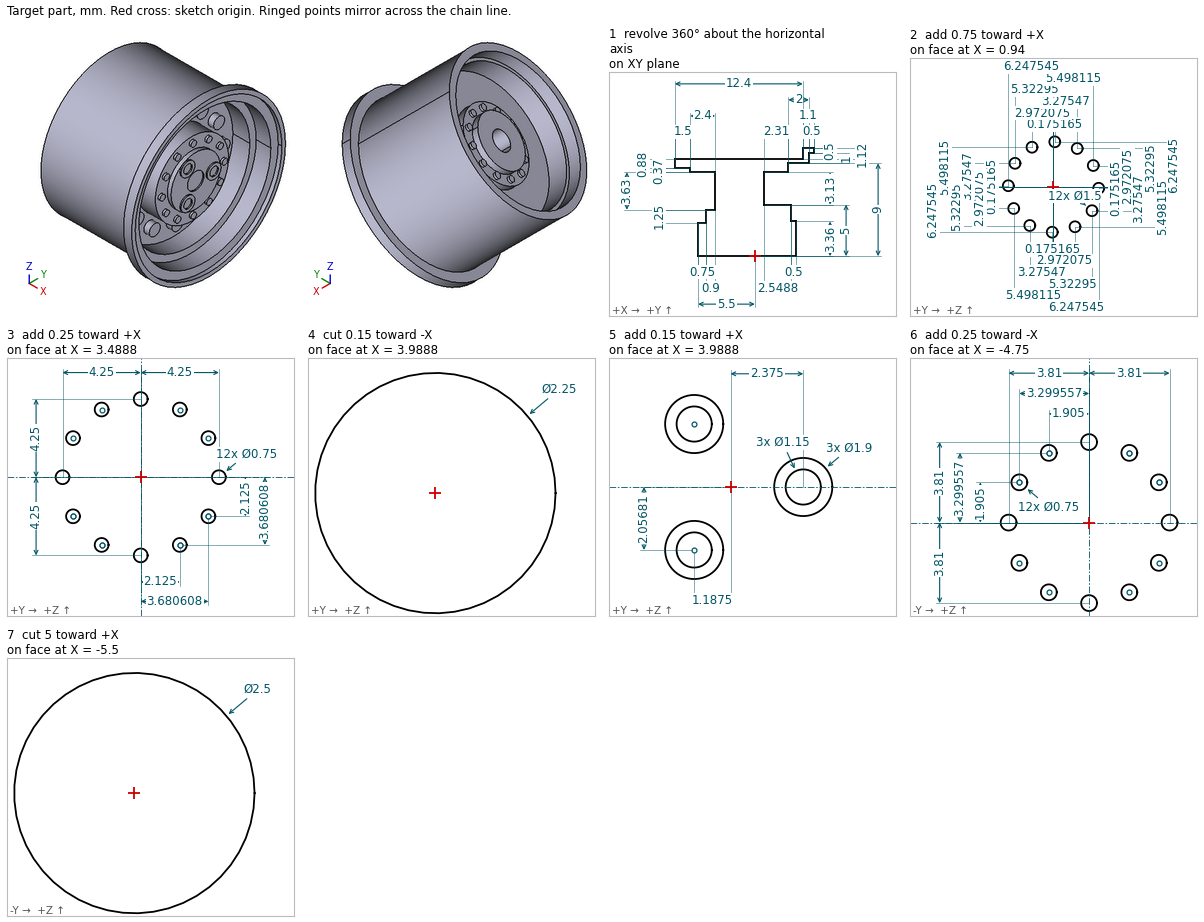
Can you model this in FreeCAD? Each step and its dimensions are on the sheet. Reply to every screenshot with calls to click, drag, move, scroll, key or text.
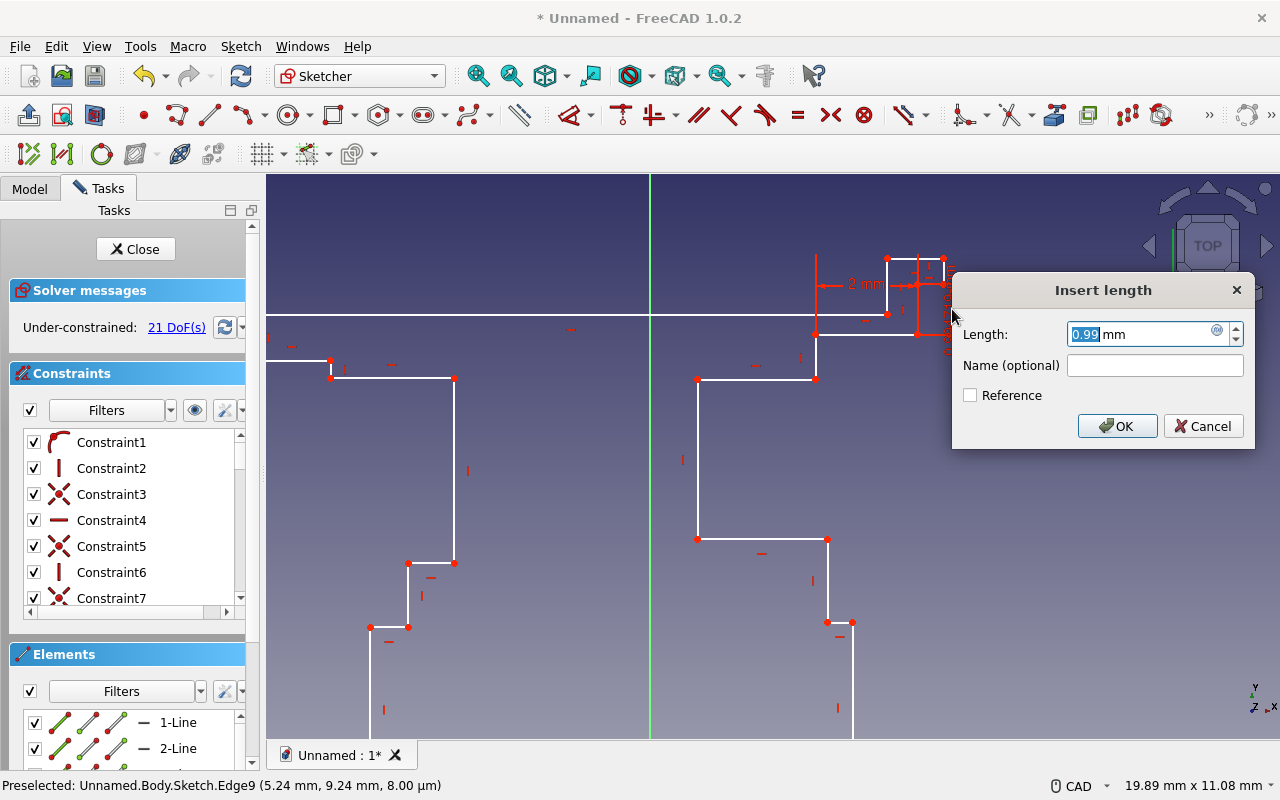
text(1)
key(Return)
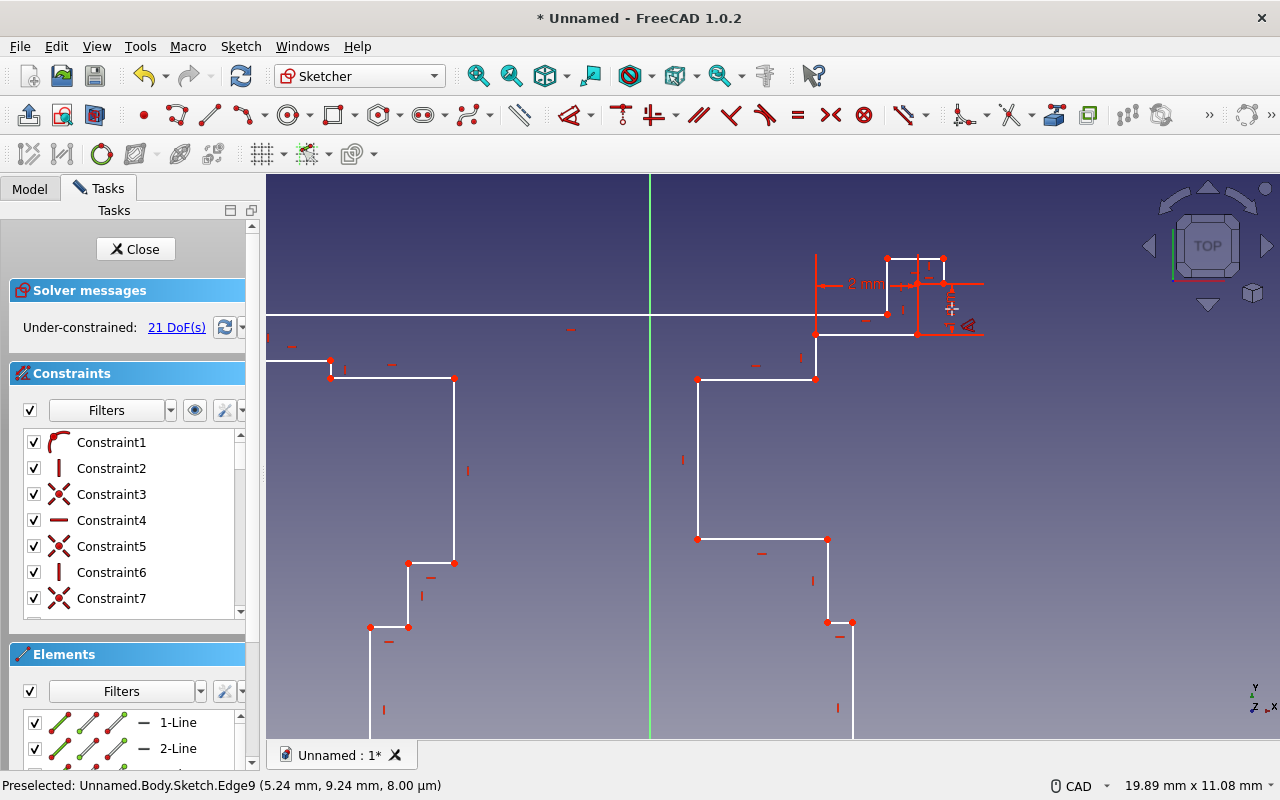
click(828, 539)
click(862, 586)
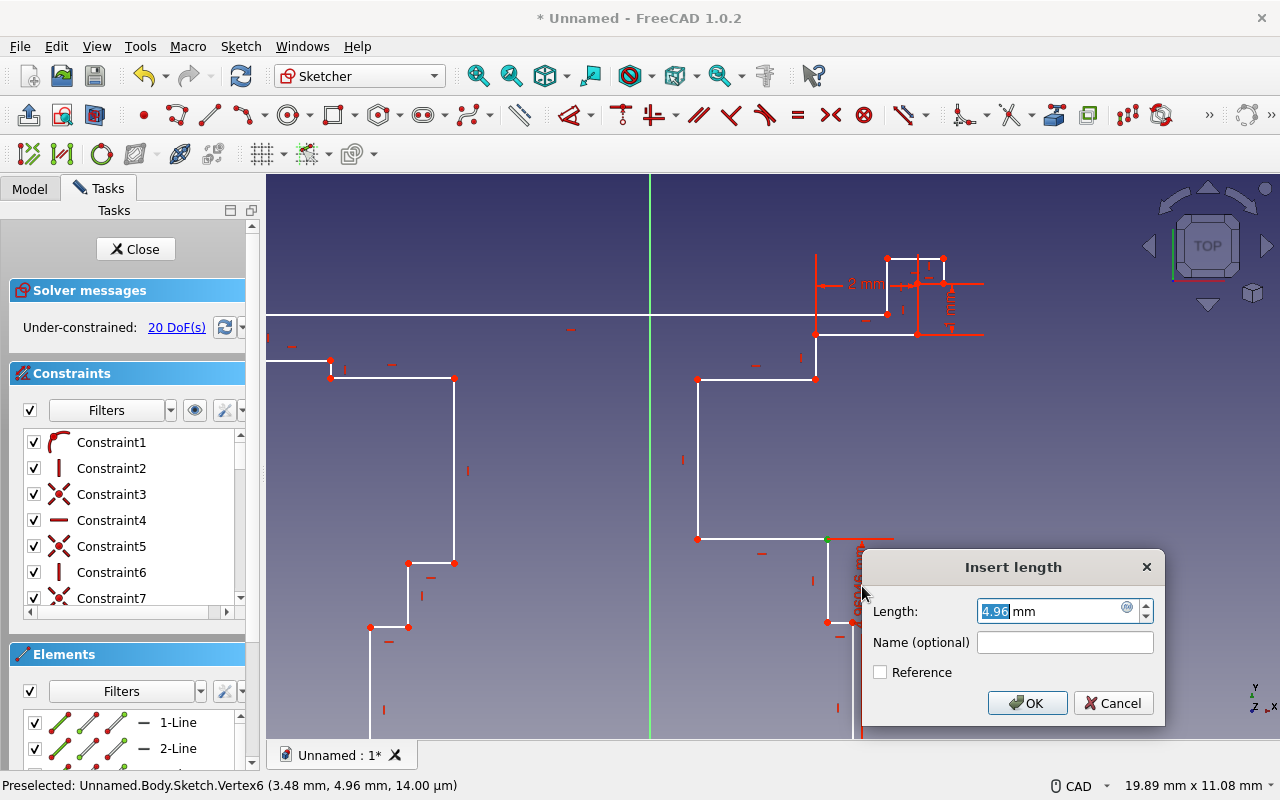
text(5)
key(Return)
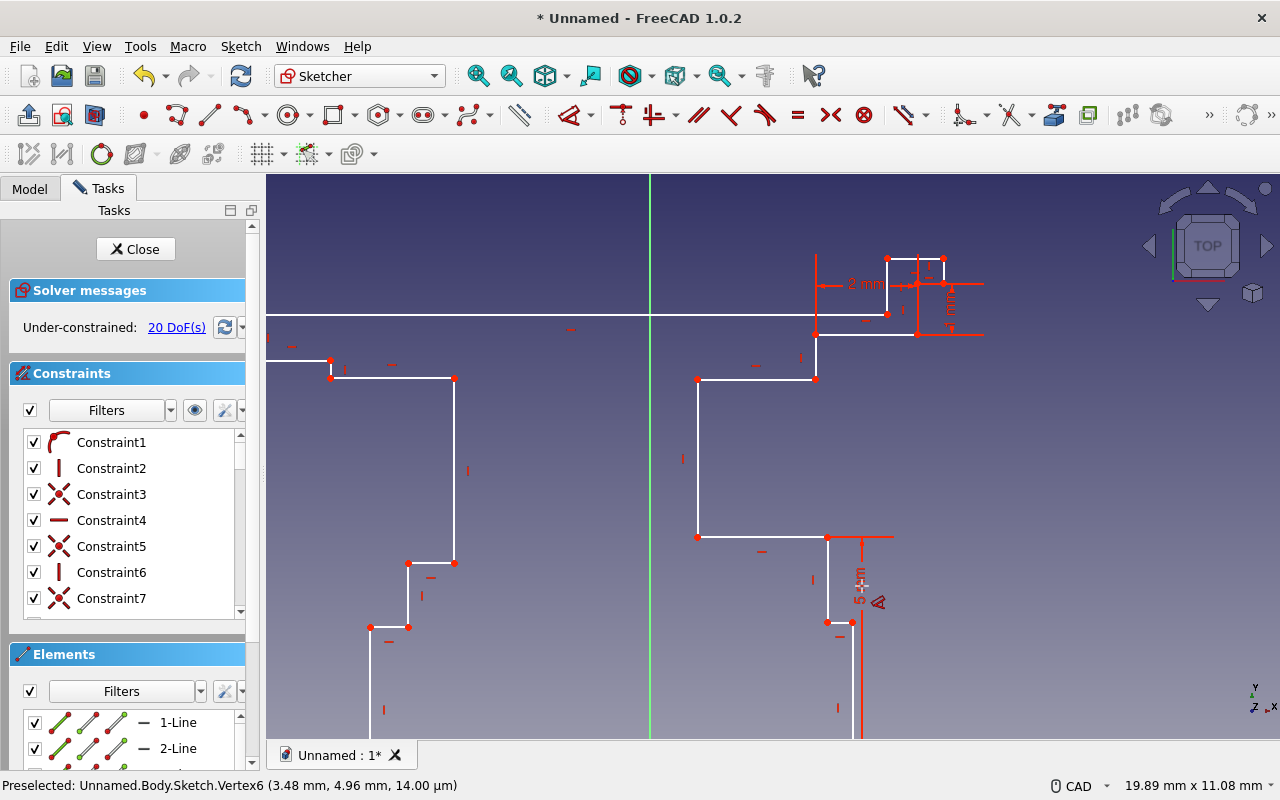
click(816, 335)
click(850, 523)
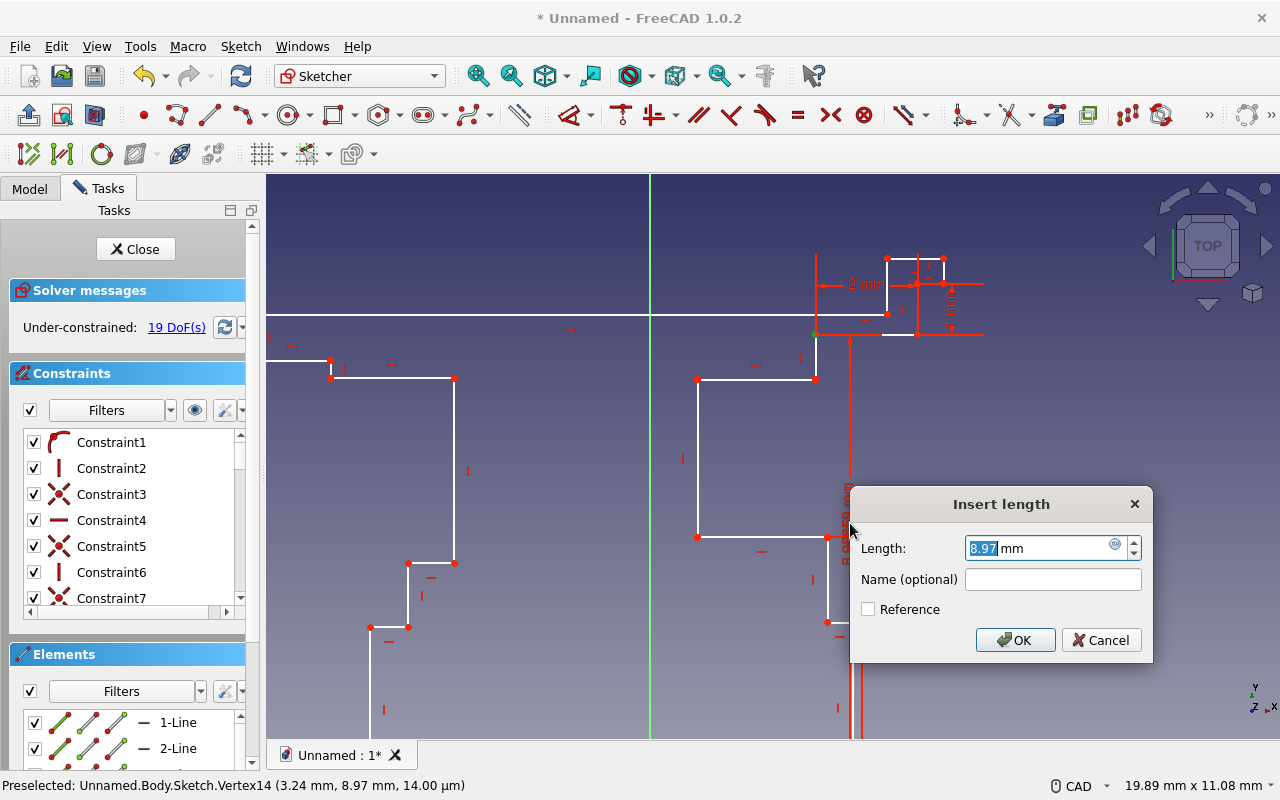
text(9)
key(Return)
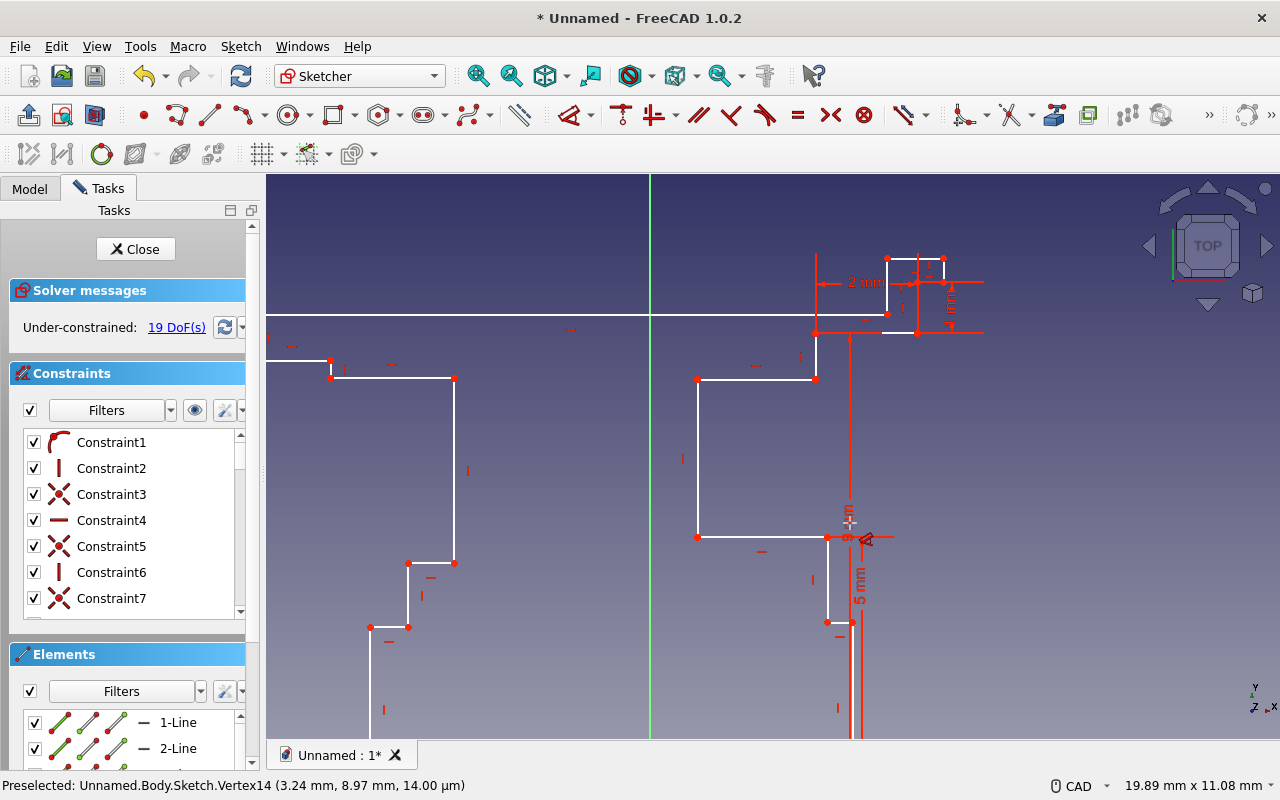
scroll(843, 623, up, 3)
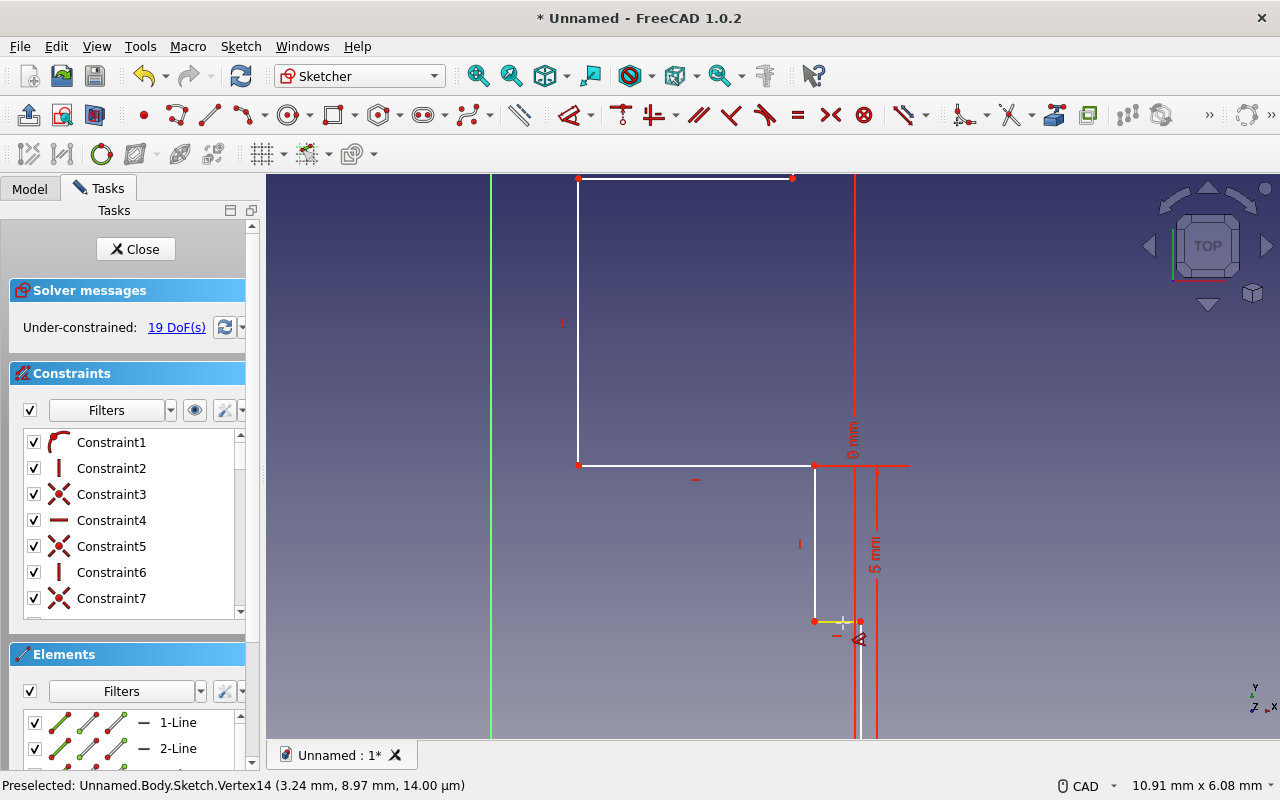
click(842, 622)
click(838, 656)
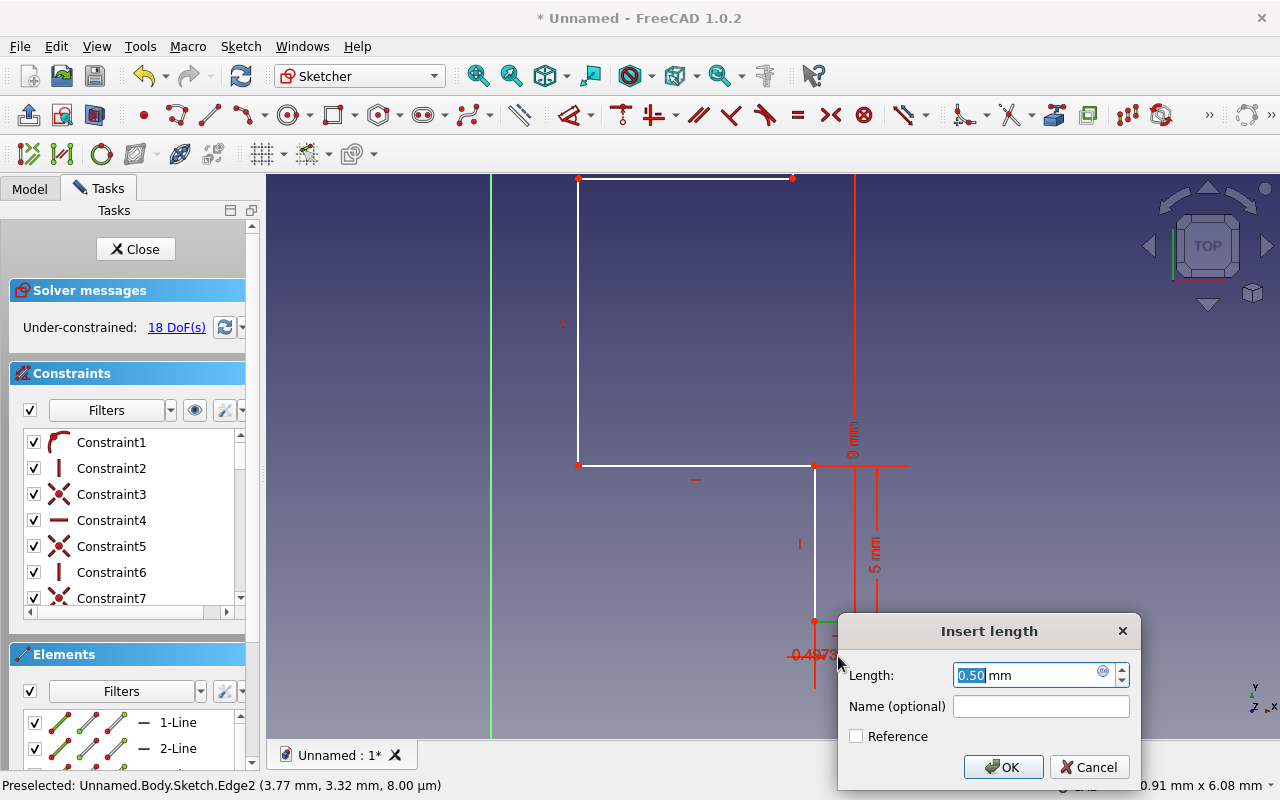
text(0.5)
key(Return)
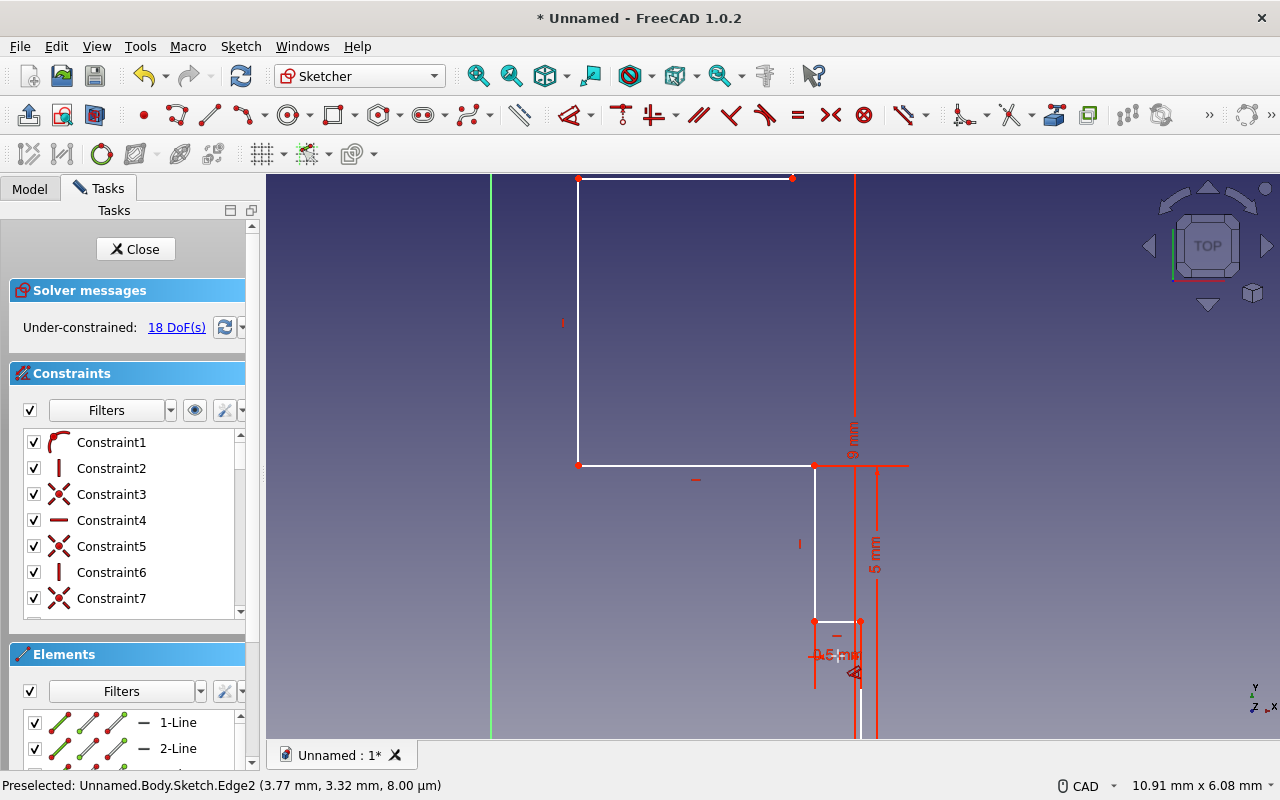
scroll(883, 465, down, 5)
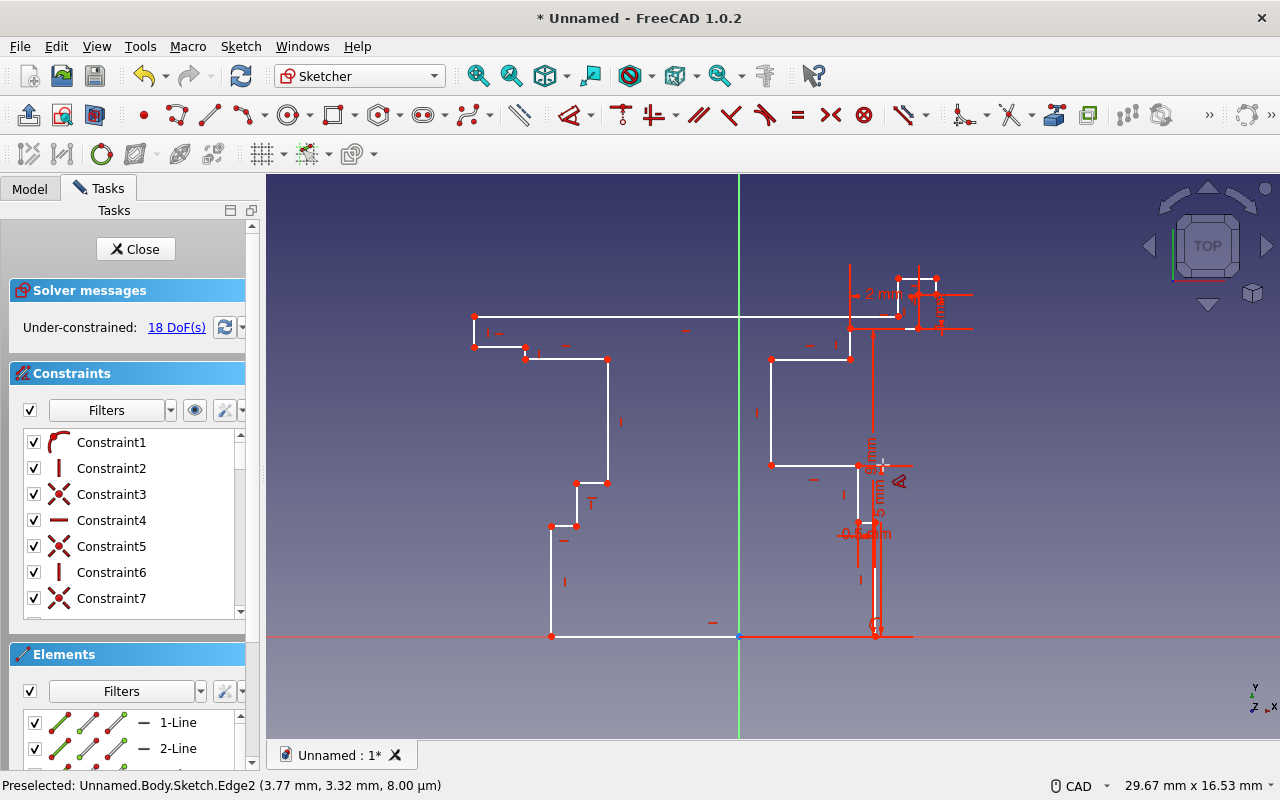
scroll(924, 295, up, 5)